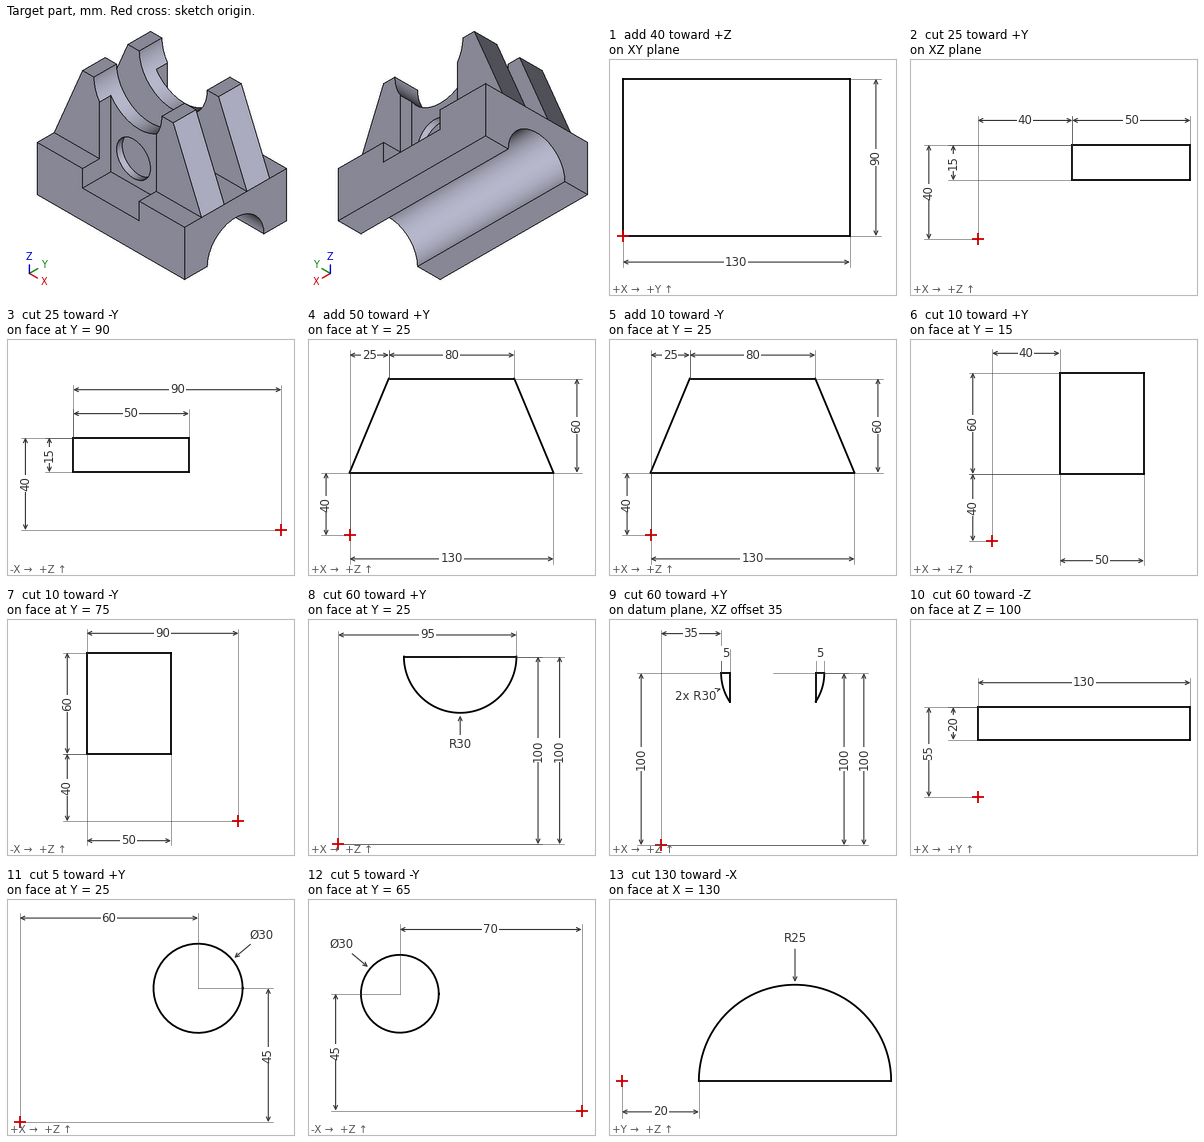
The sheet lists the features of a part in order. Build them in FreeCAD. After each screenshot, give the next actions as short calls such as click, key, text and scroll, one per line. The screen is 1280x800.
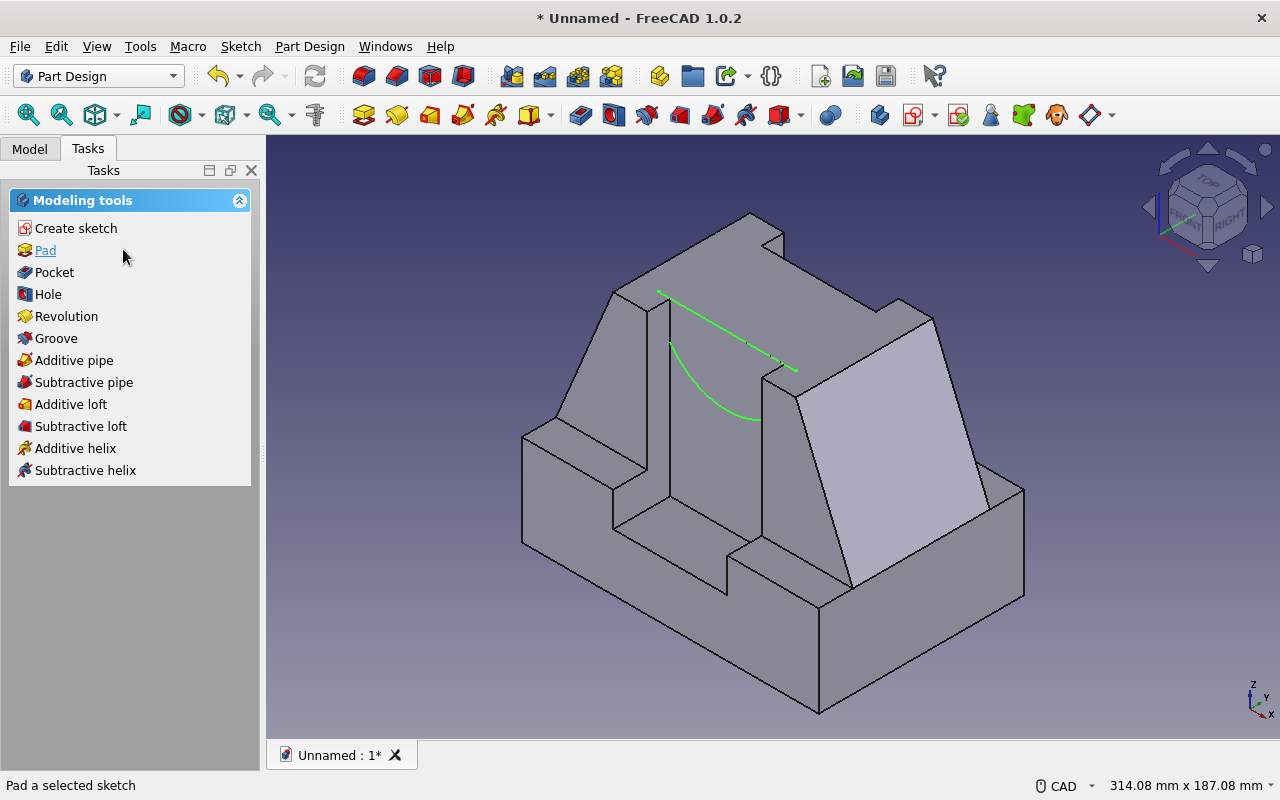
click(581, 116)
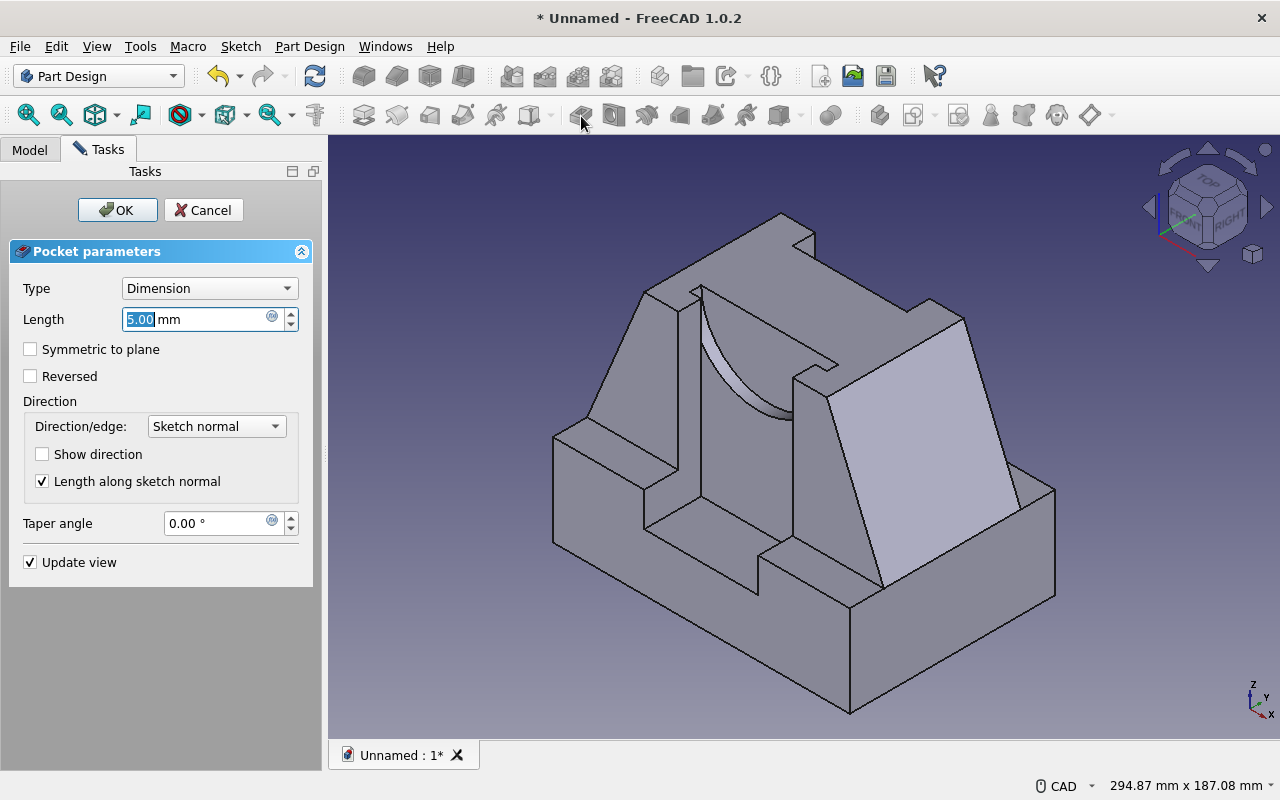
text(60)
key(Tab)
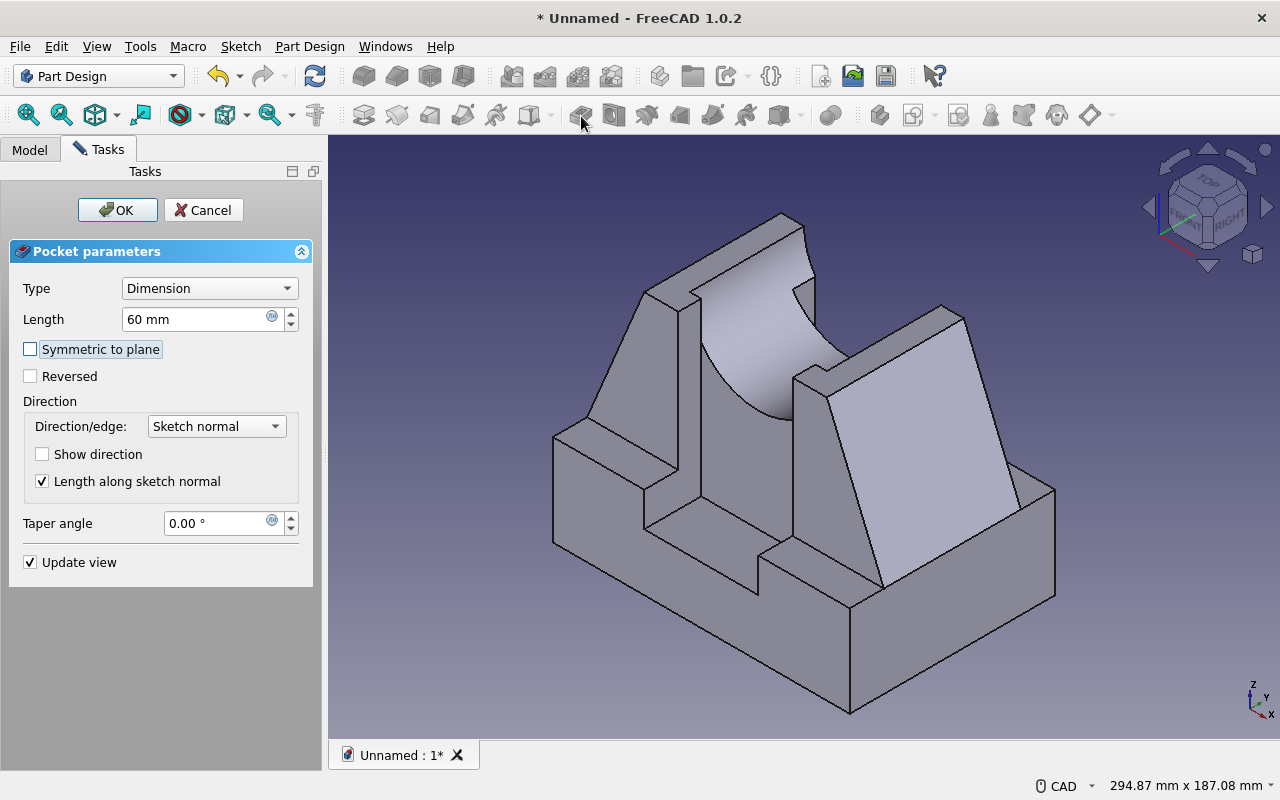
click(118, 210)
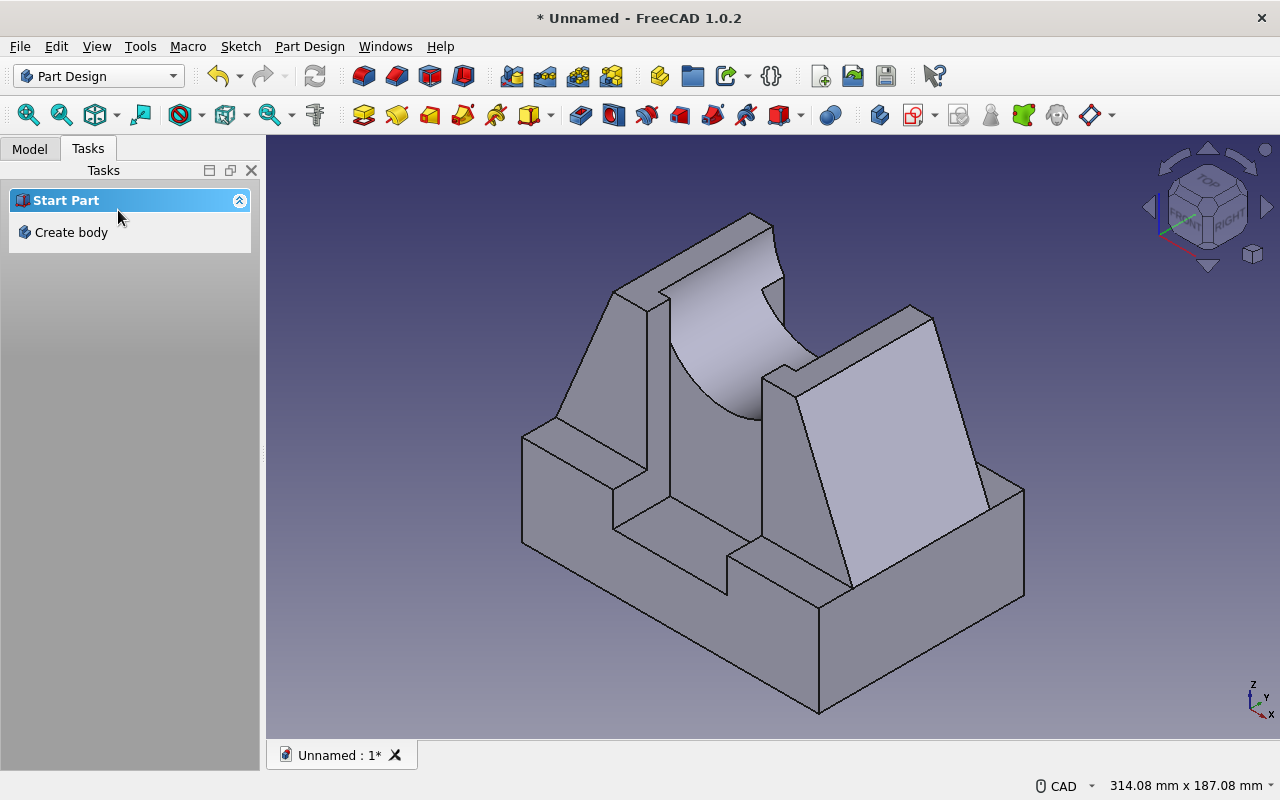
click(30, 148)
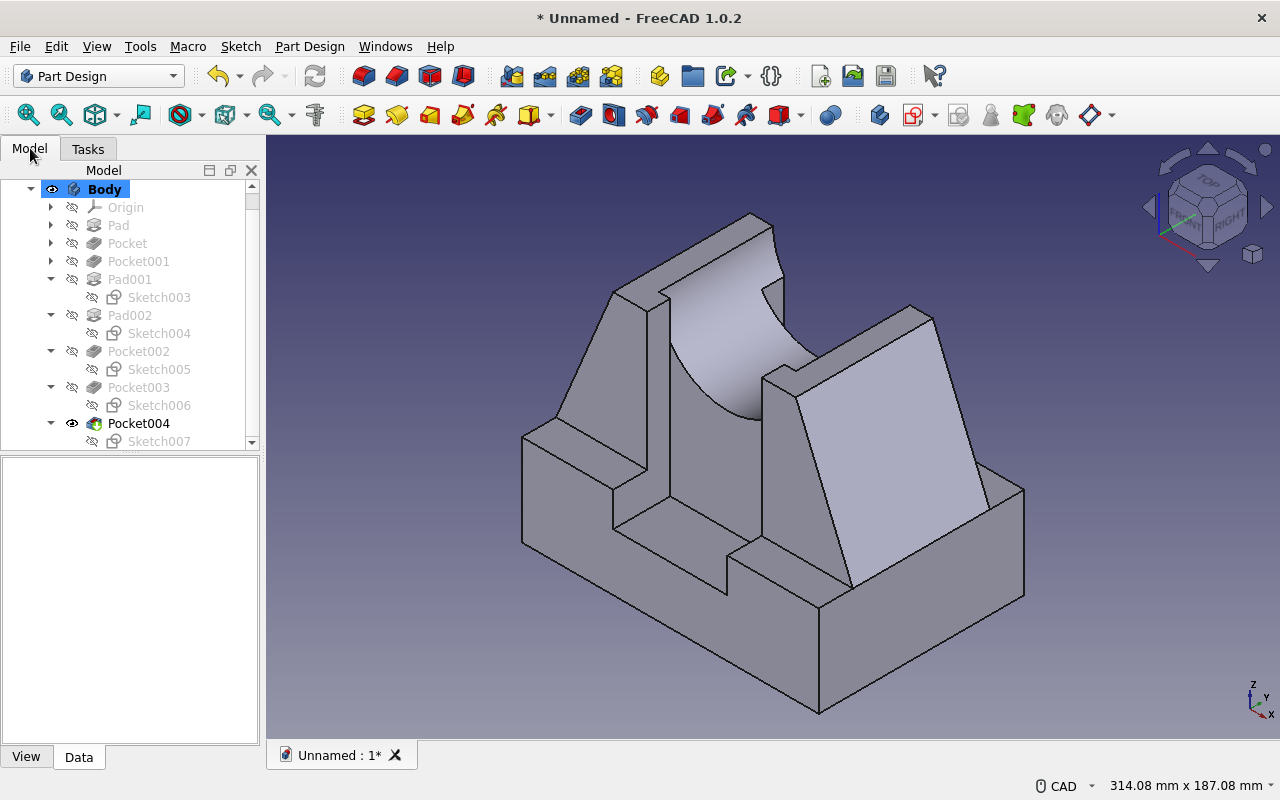
click(51, 207)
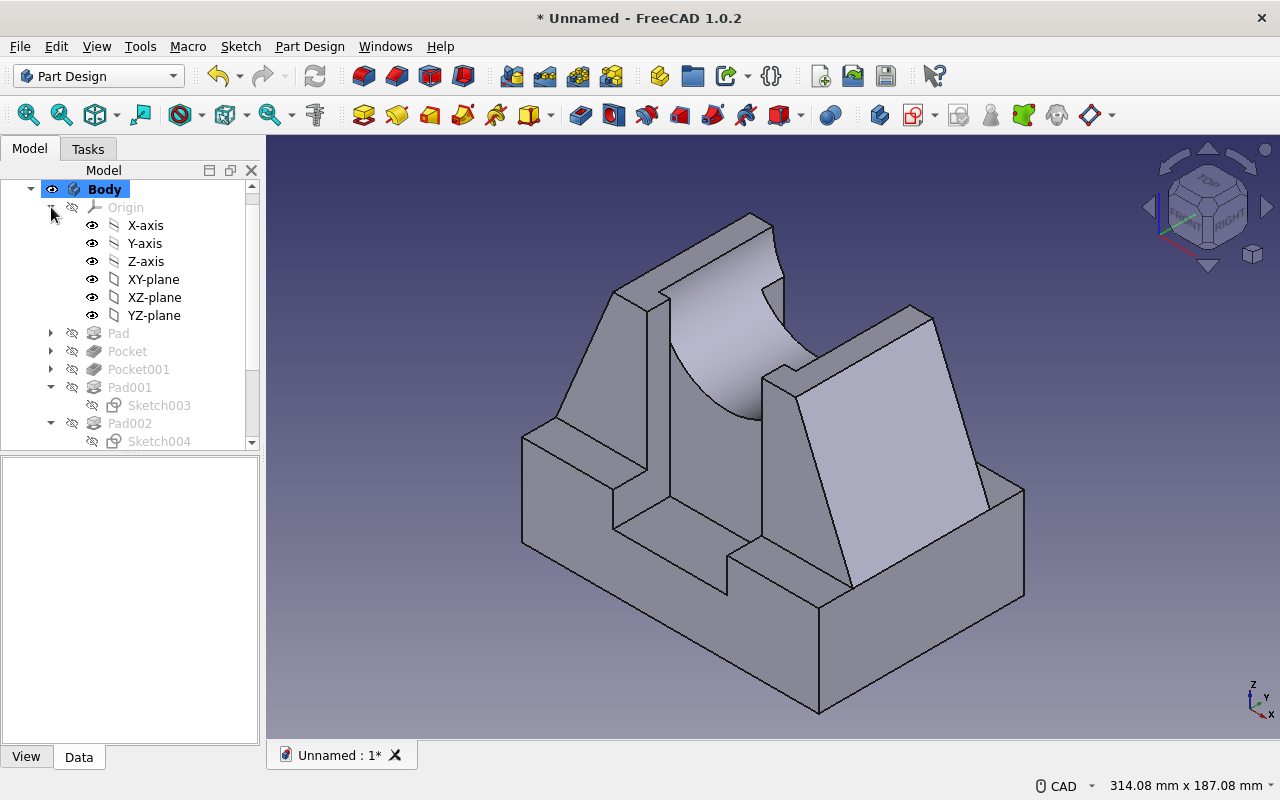
click(137, 297)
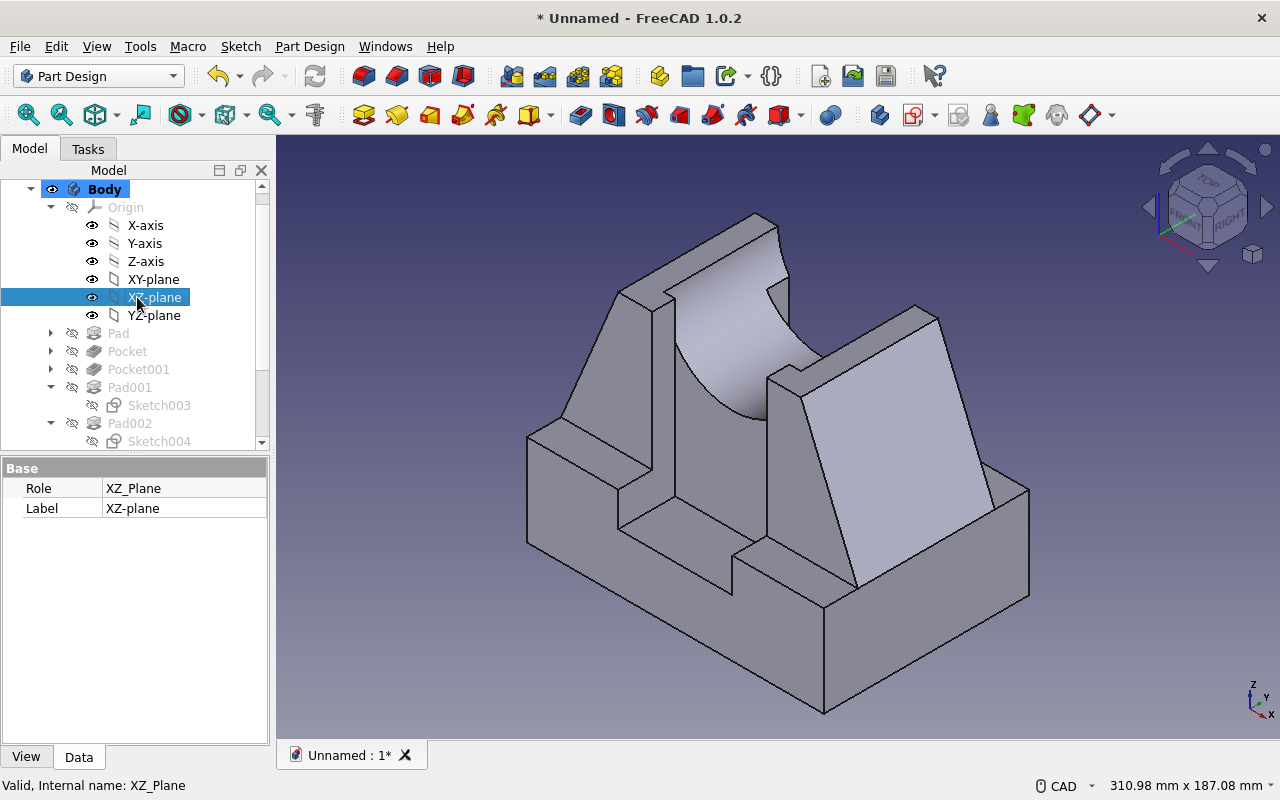
click(1090, 116)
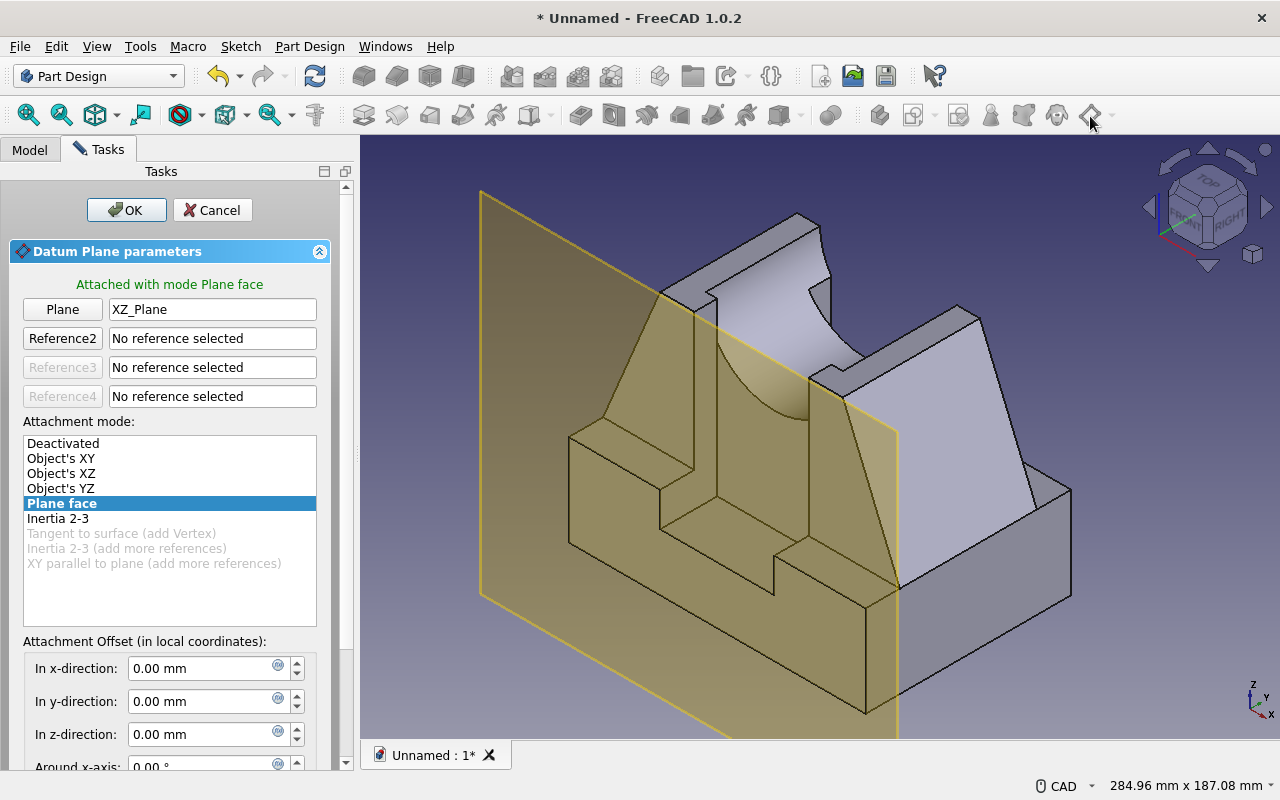
triple_click(210, 734)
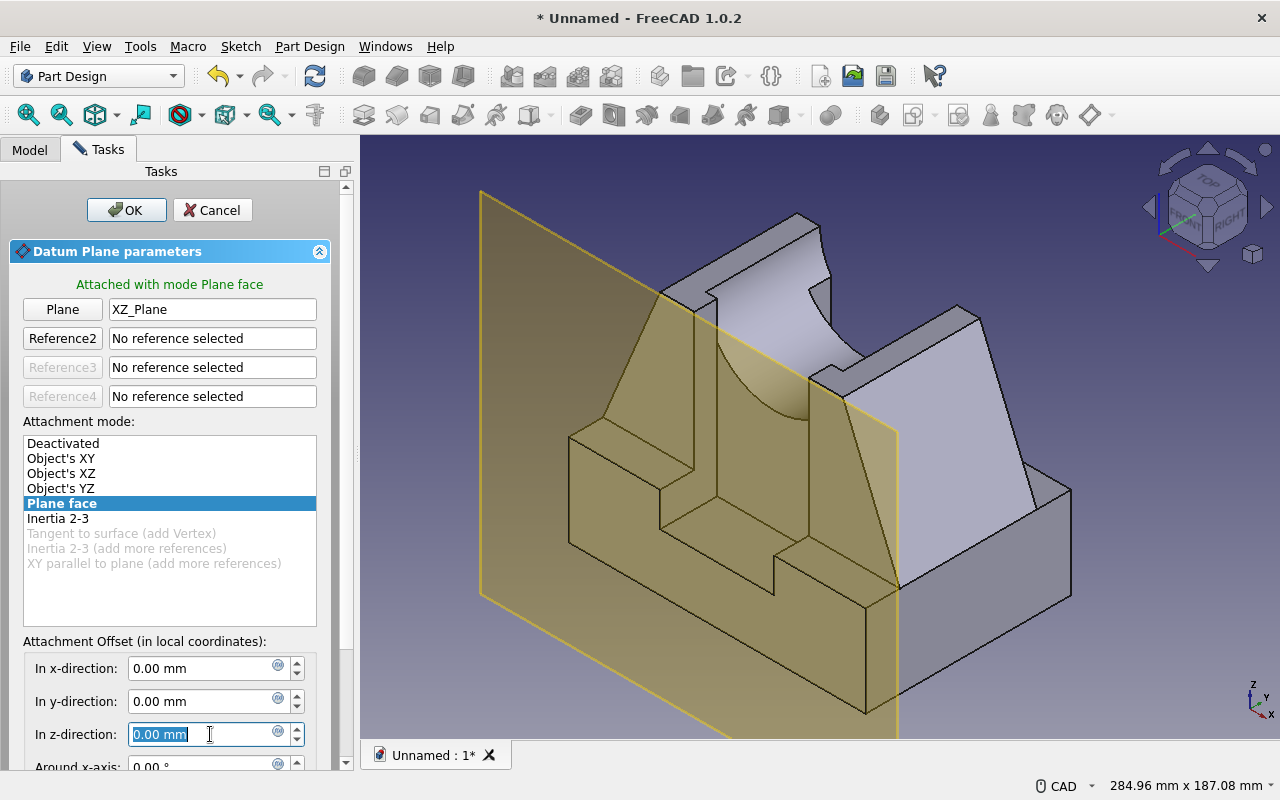
text(35)
key(Tab)